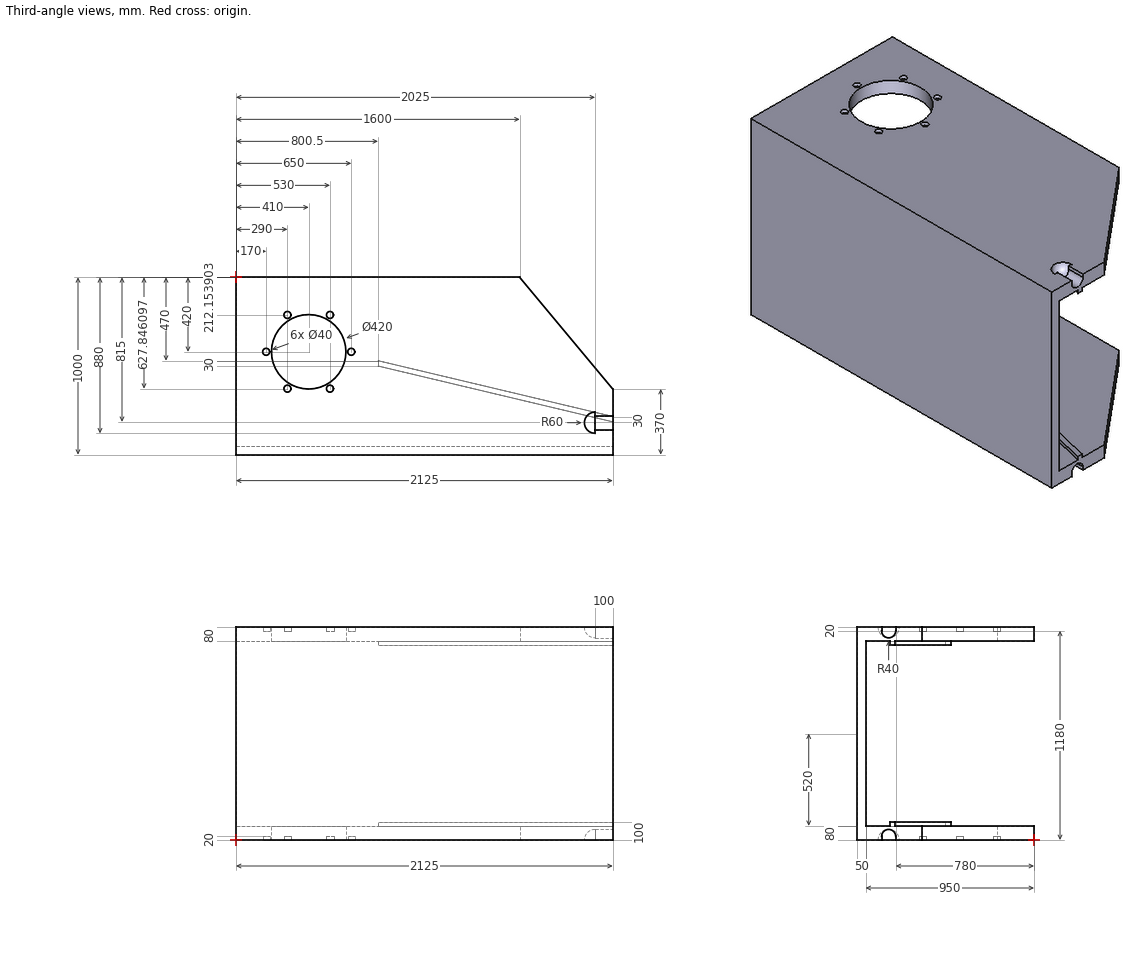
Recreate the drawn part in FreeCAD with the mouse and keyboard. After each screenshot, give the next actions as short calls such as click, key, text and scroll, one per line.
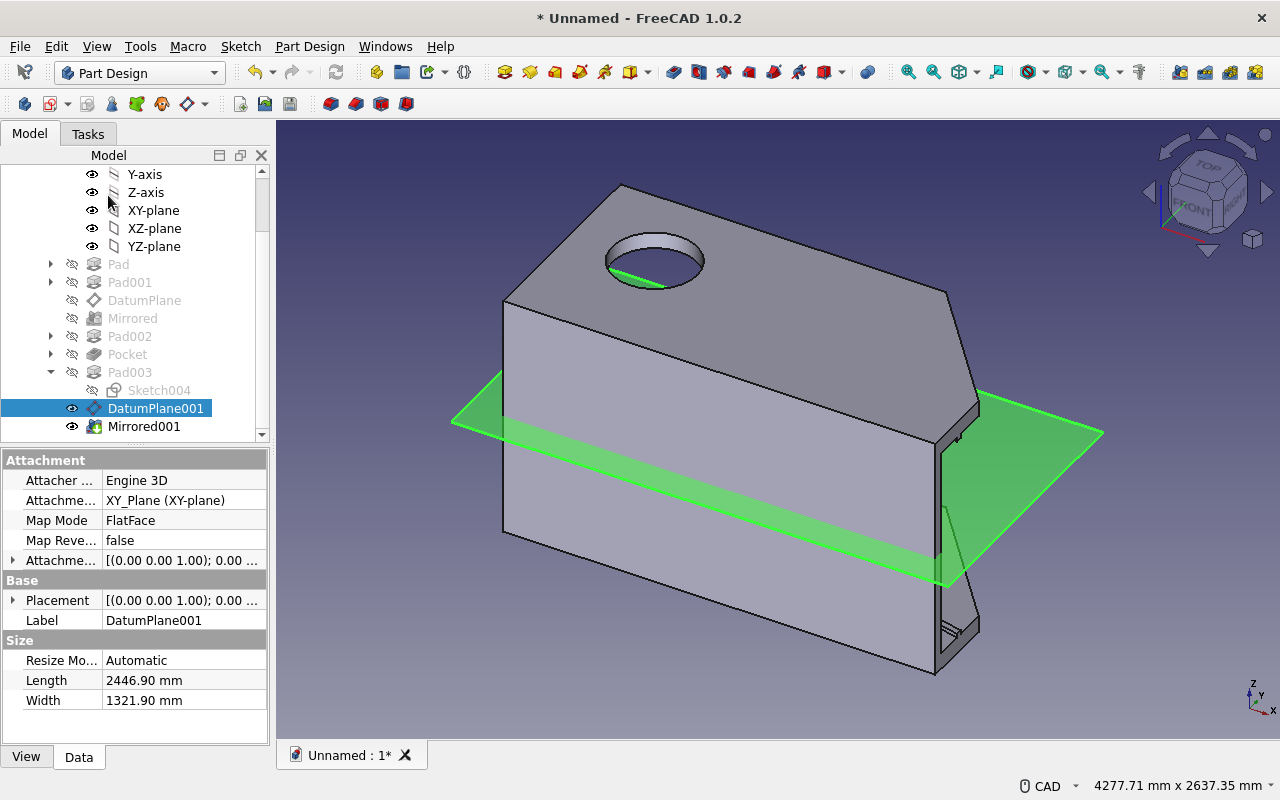
click(117, 408)
key(space)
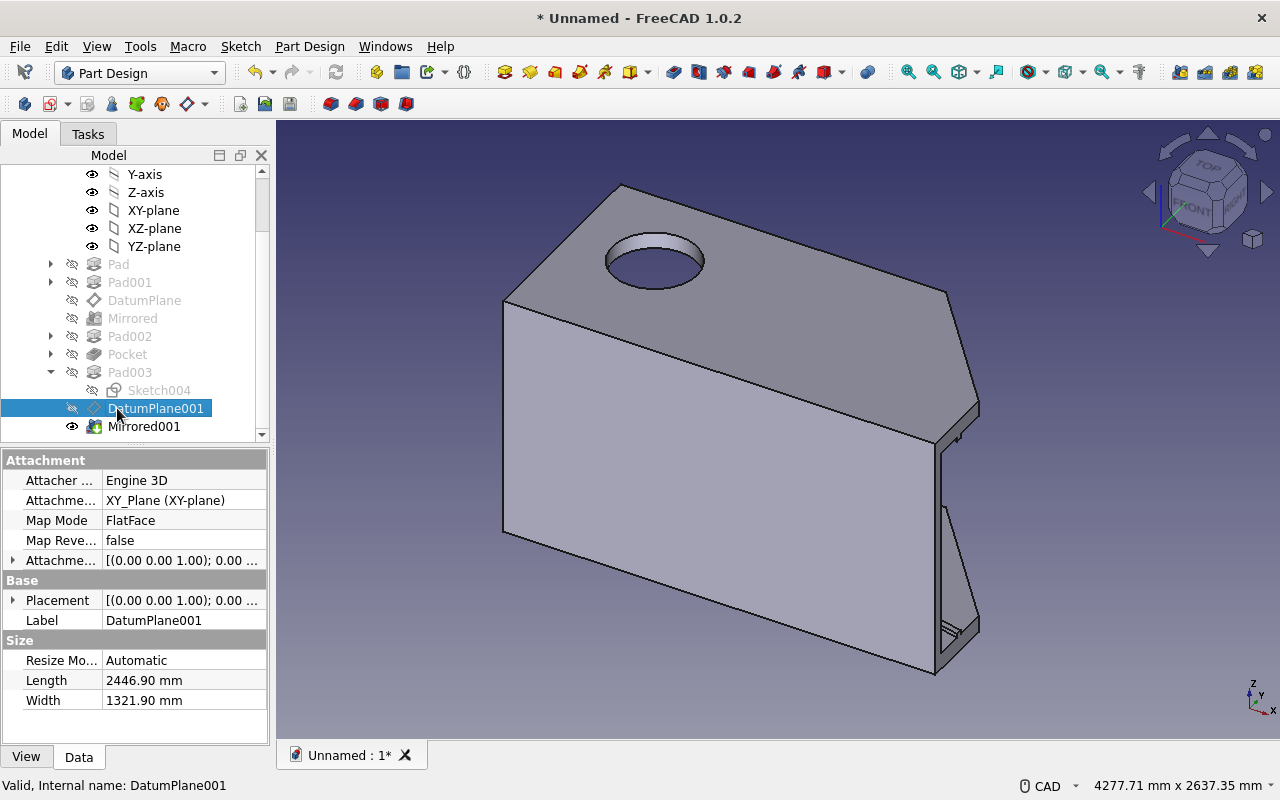
key(5)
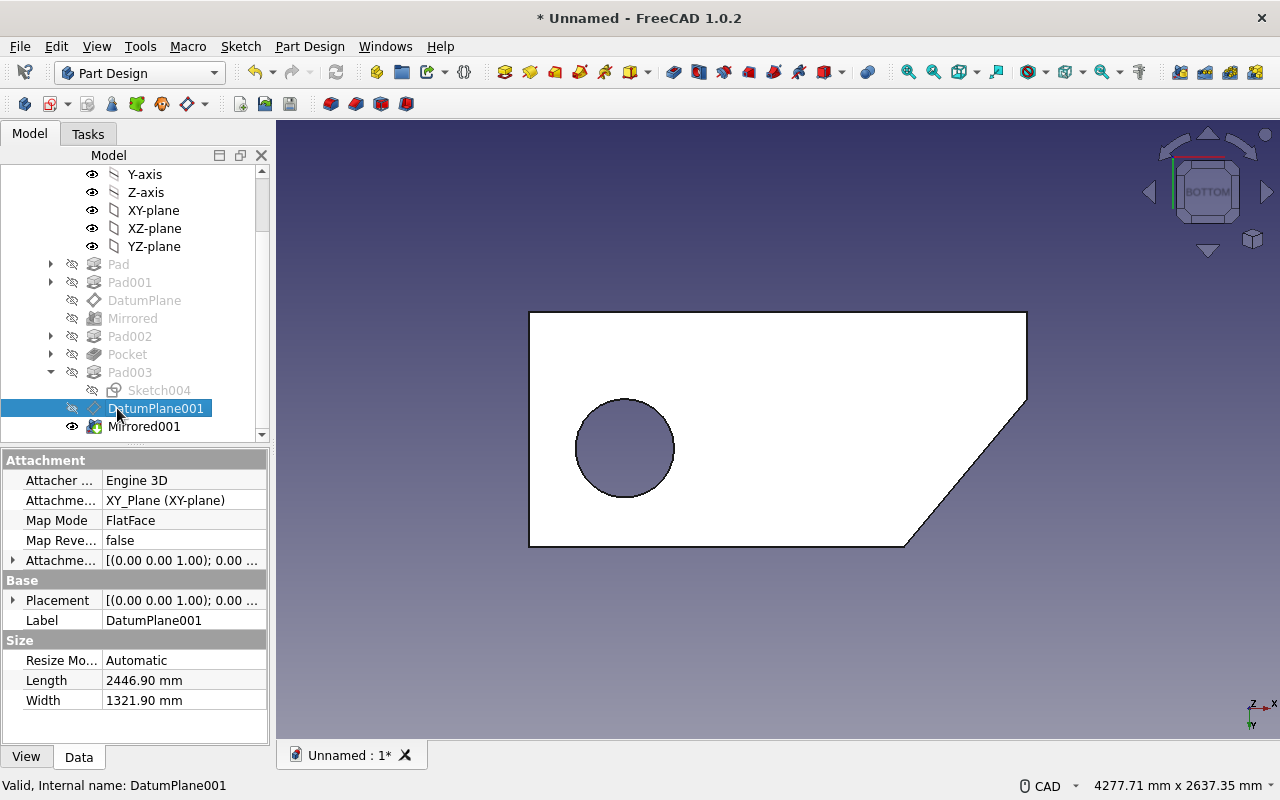
click(849, 429)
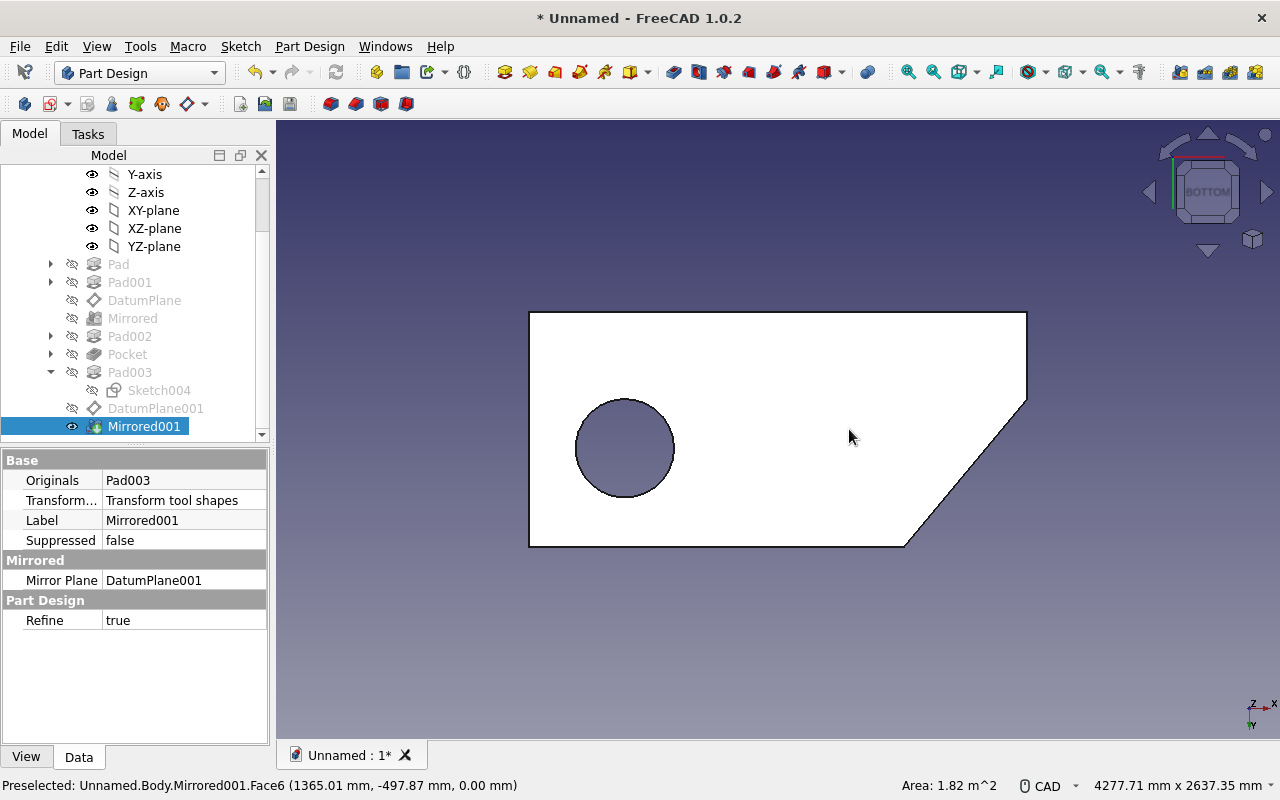
click(50, 104)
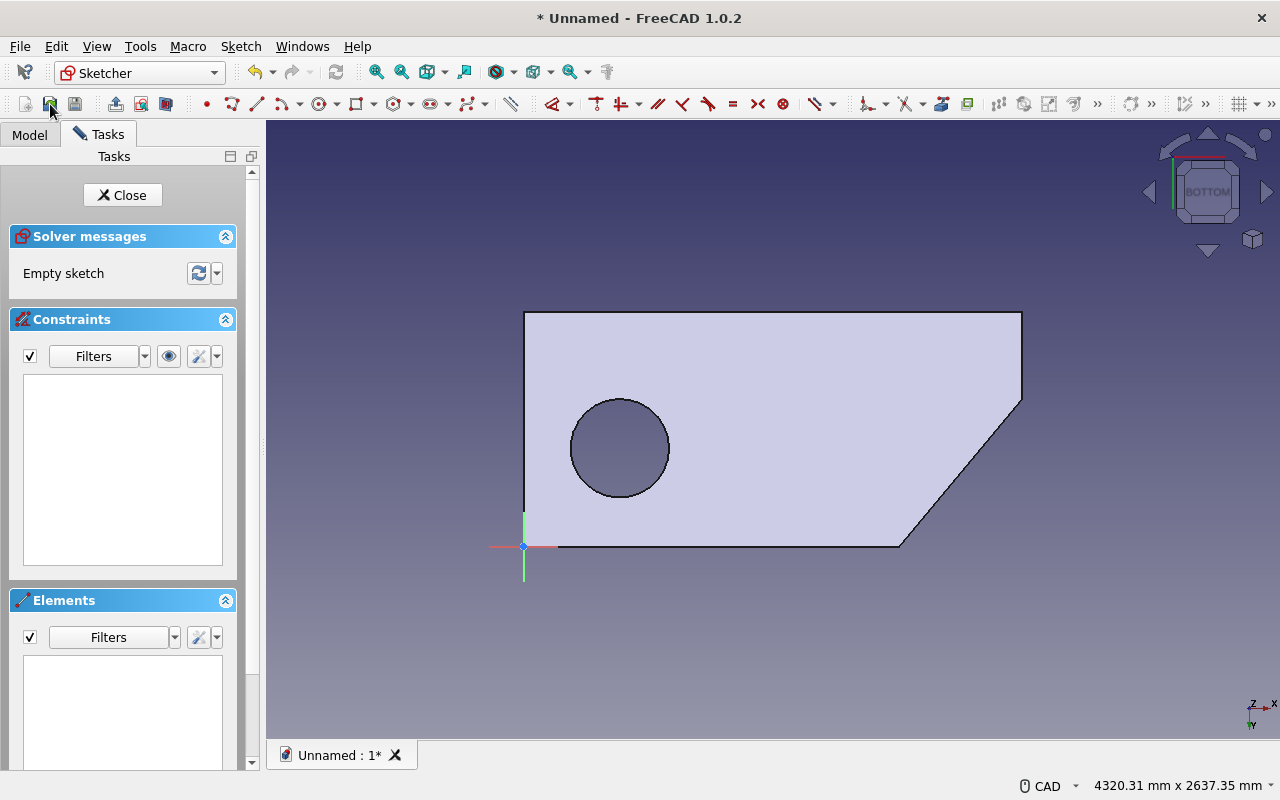
scroll(543, 495, up, 5)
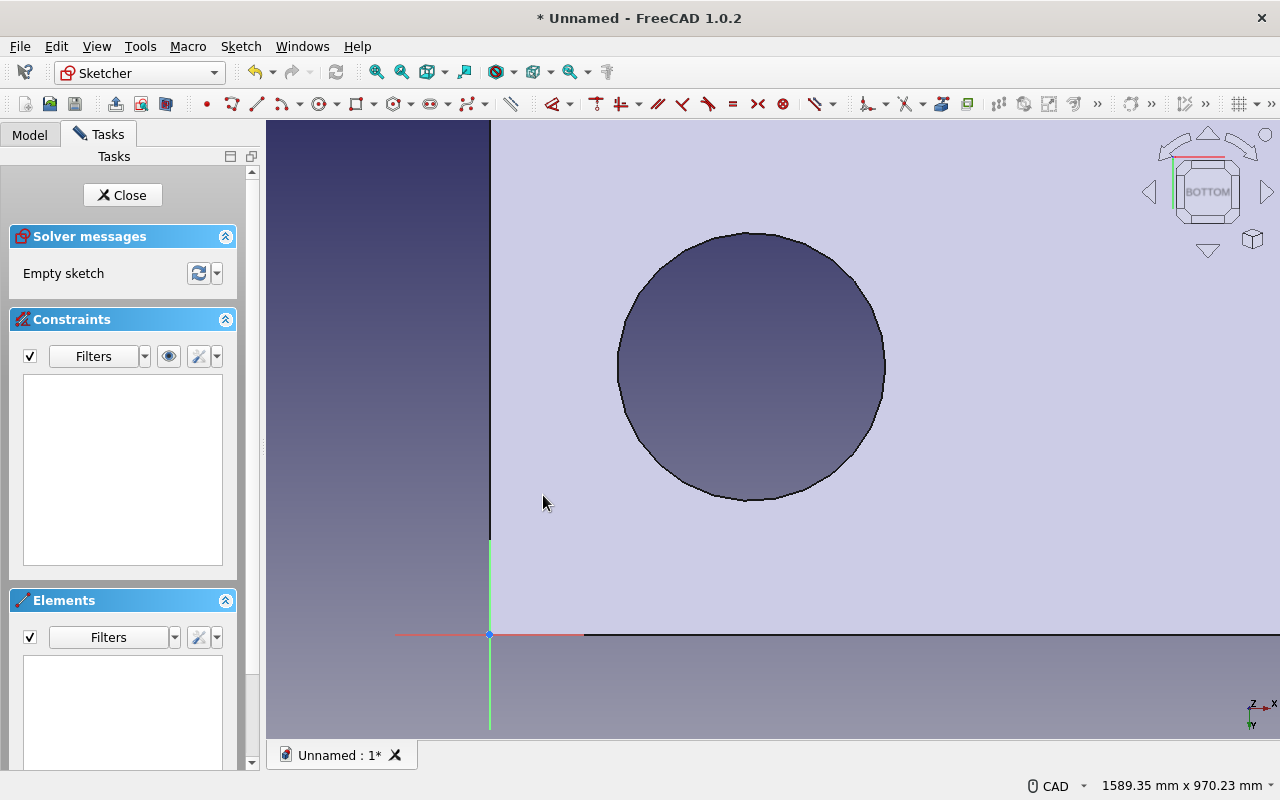
key(g)
key(c)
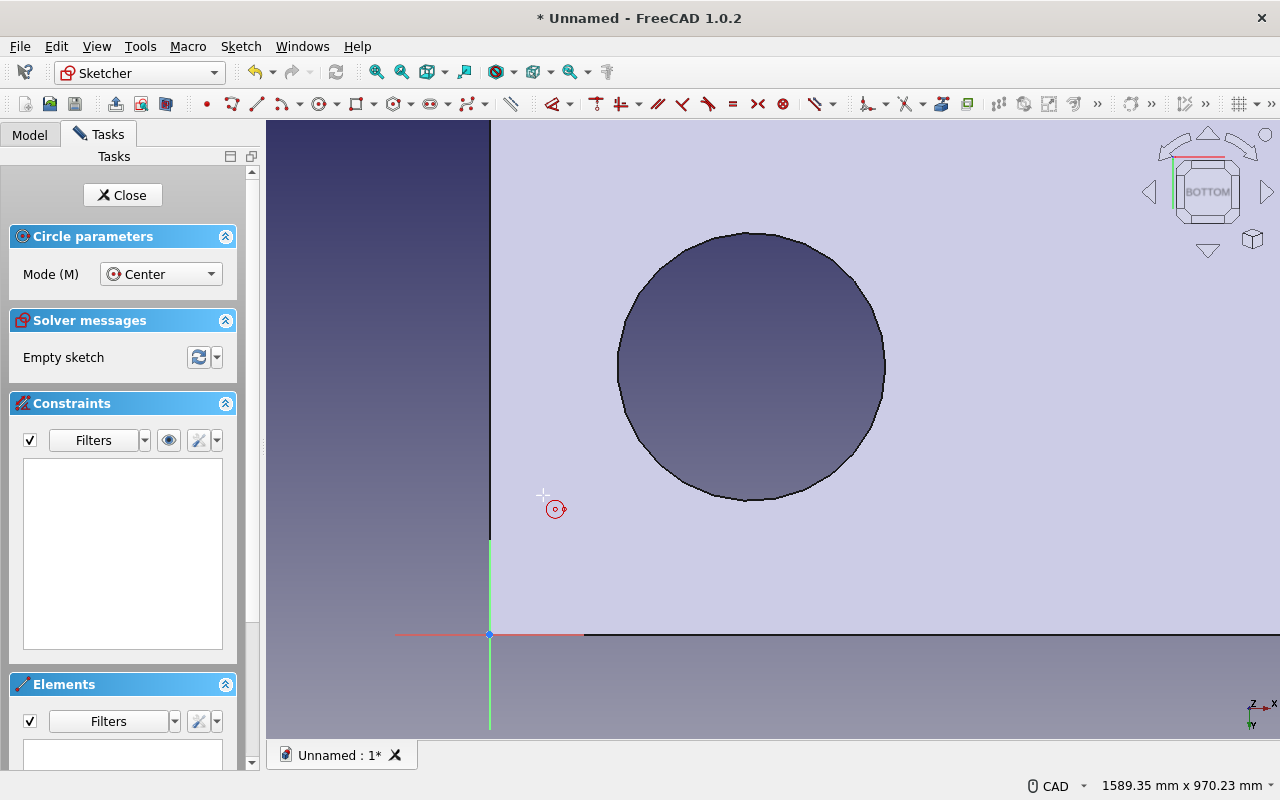
scroll(598, 367, up, 3)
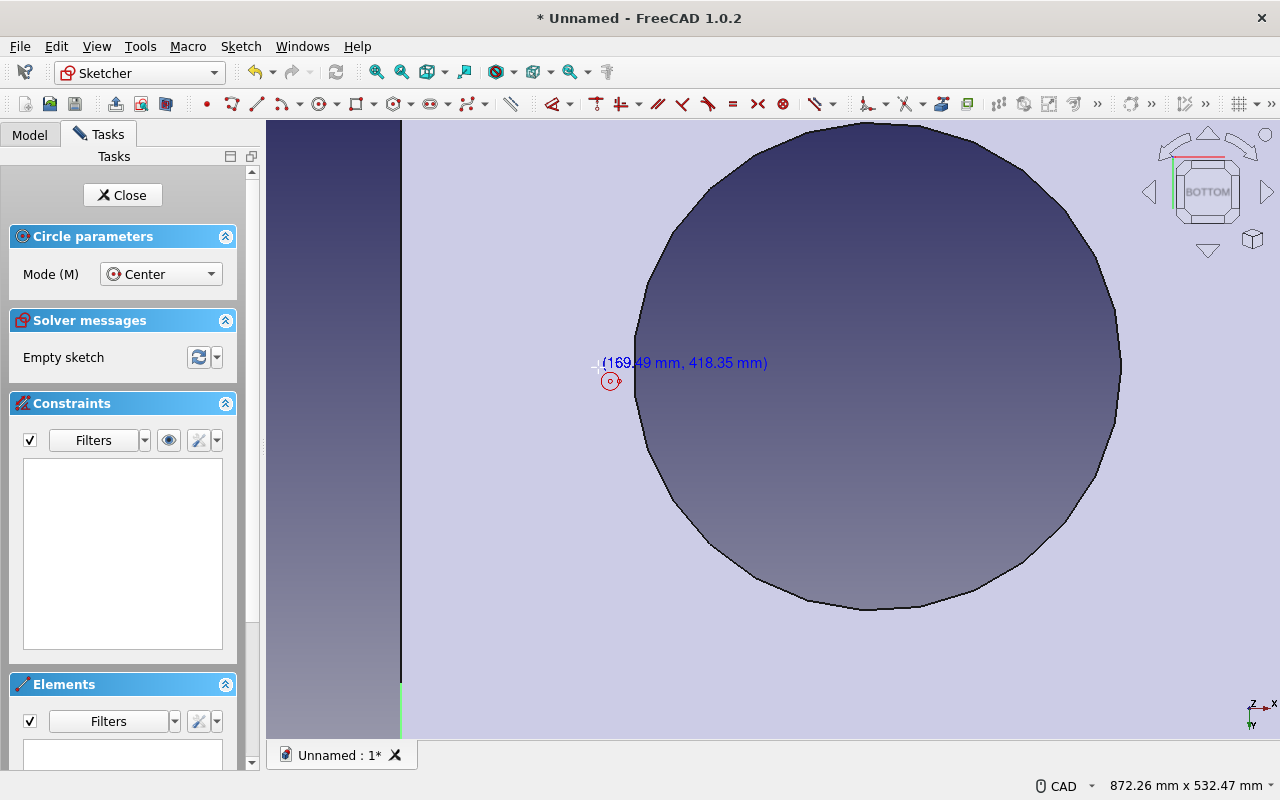
click(598, 367)
click(615, 350)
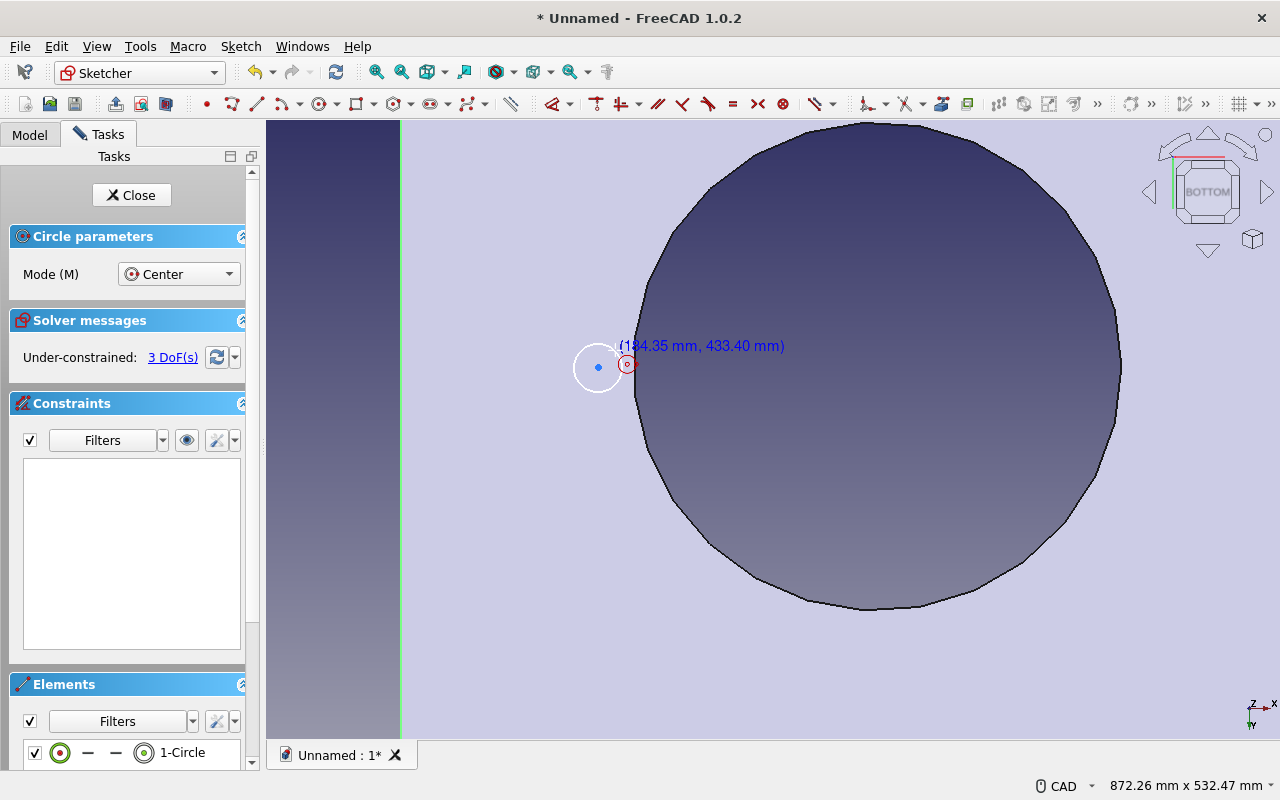
scroll(600, 370, down, 3)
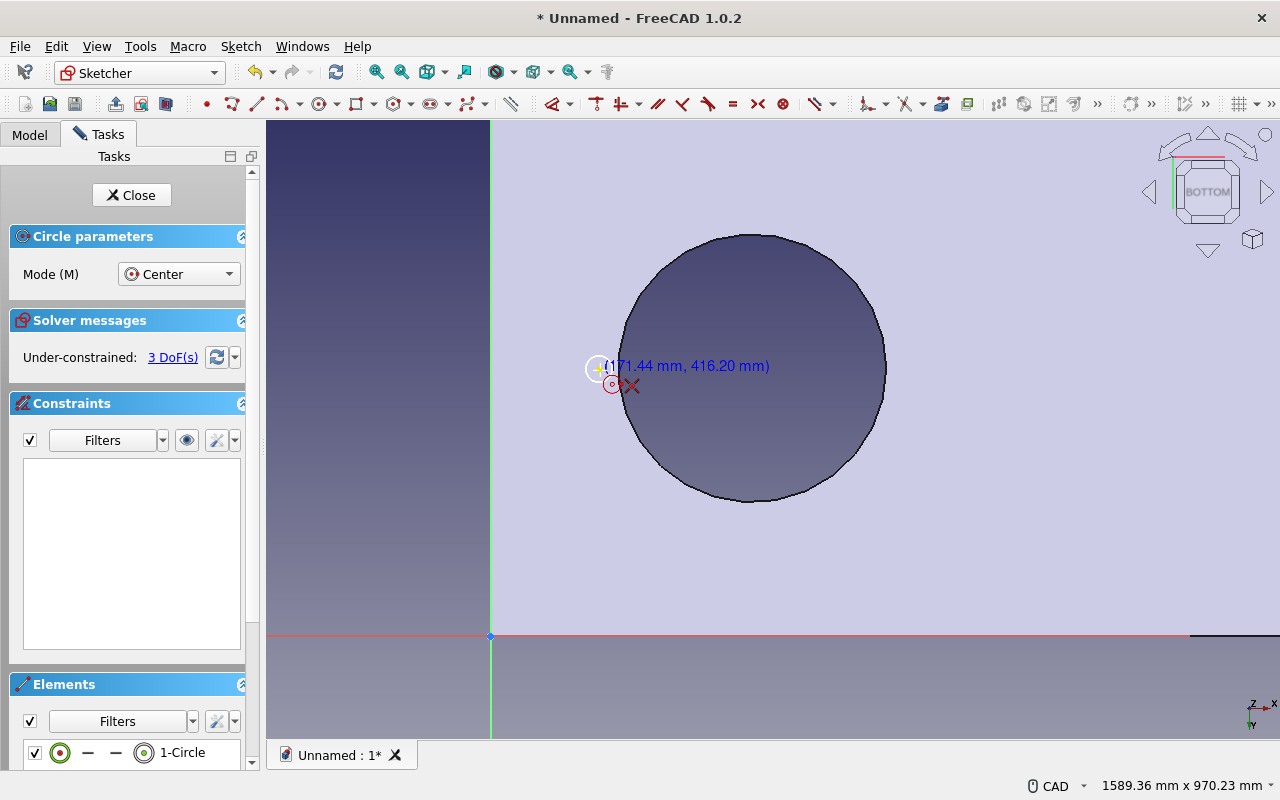
scroll(676, 236, up, 3)